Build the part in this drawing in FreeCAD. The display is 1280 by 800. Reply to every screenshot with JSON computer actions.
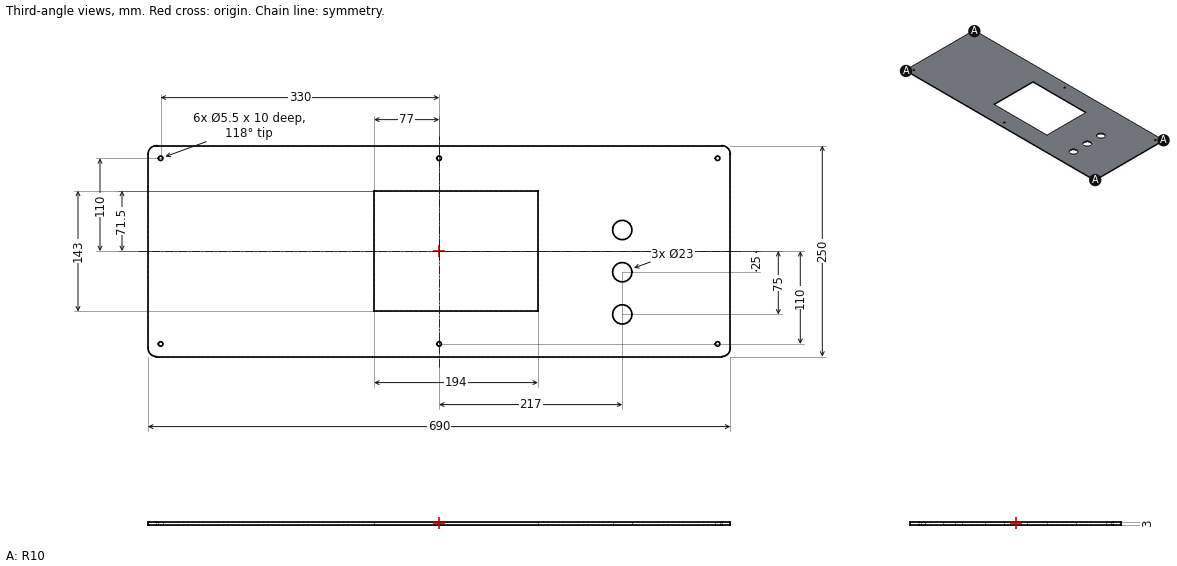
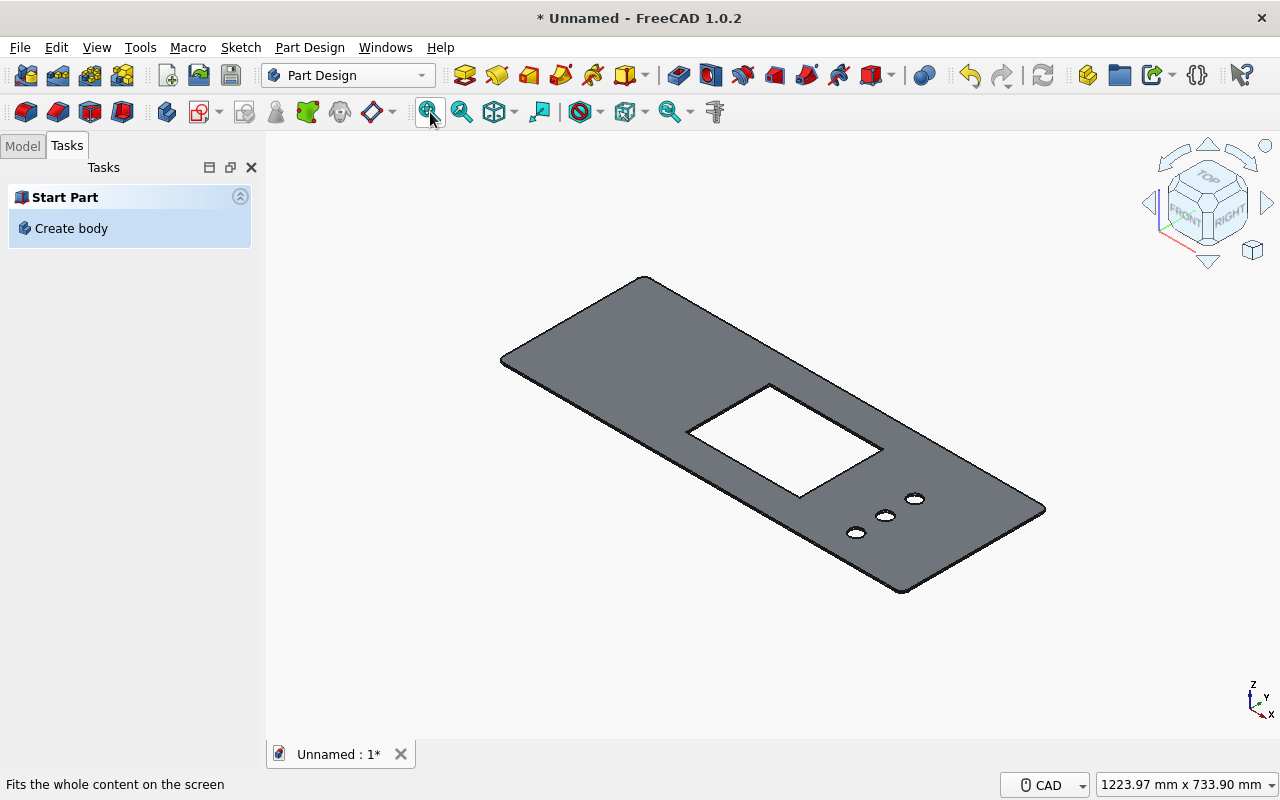
{"action": "left_click", "coordinate": [658, 366]}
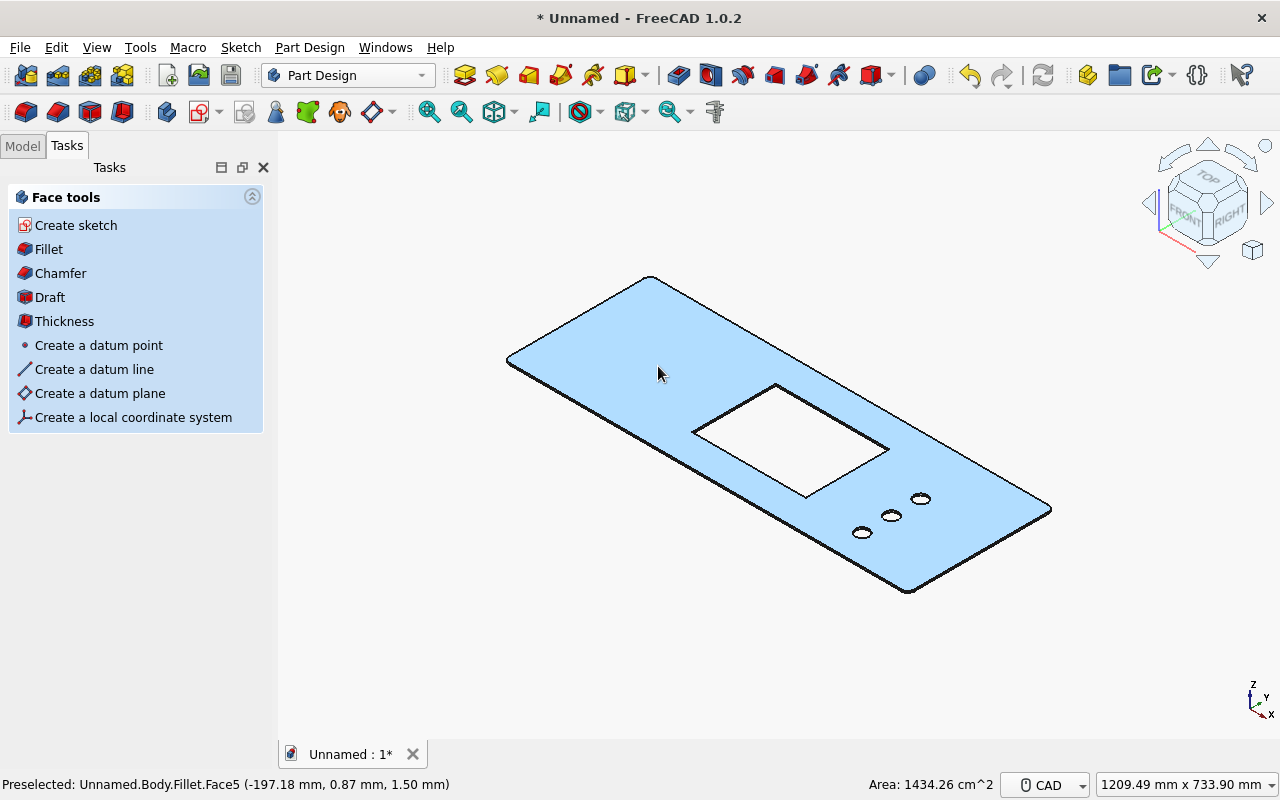
{"action": "left_click", "coordinate": [200, 112]}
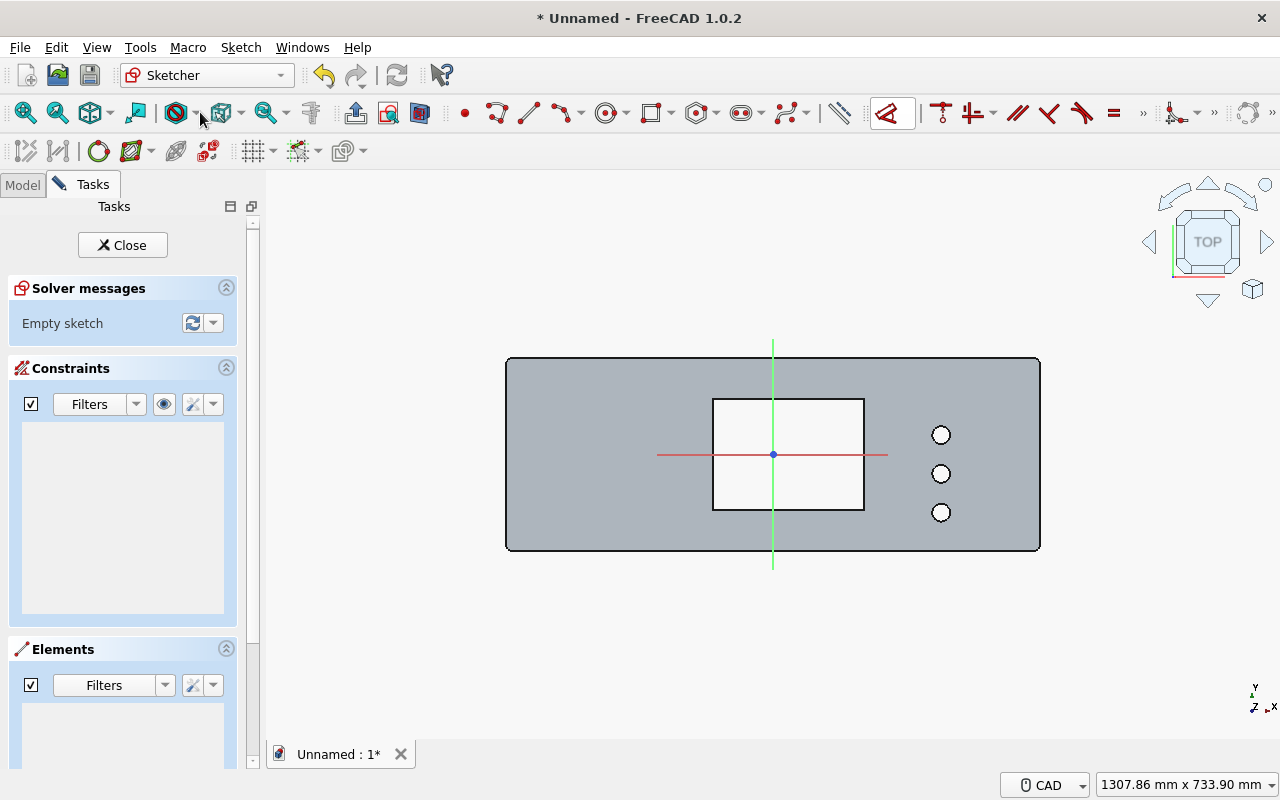
{"action": "left_click", "coordinate": [606, 114]}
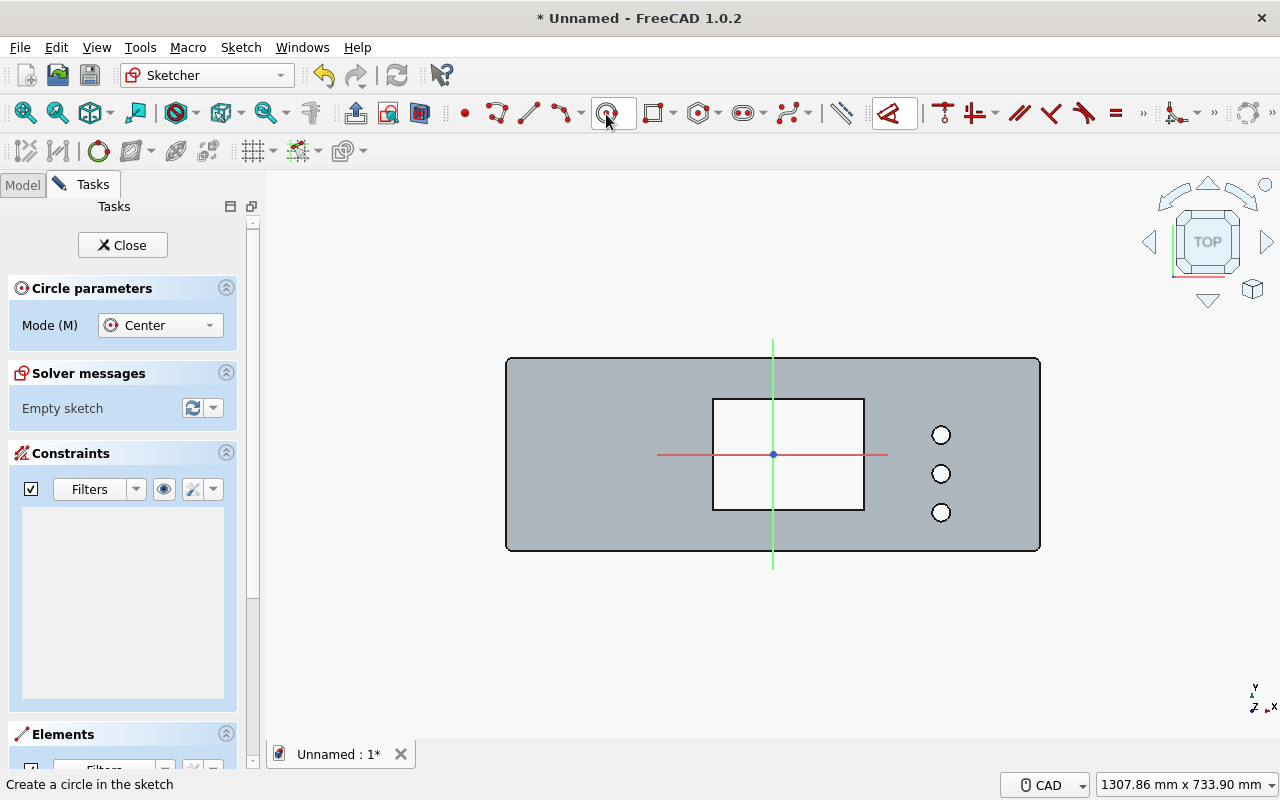
{"action": "scroll", "coordinate": [517, 369], "scroll_direction": "up", "scroll_amount": 12}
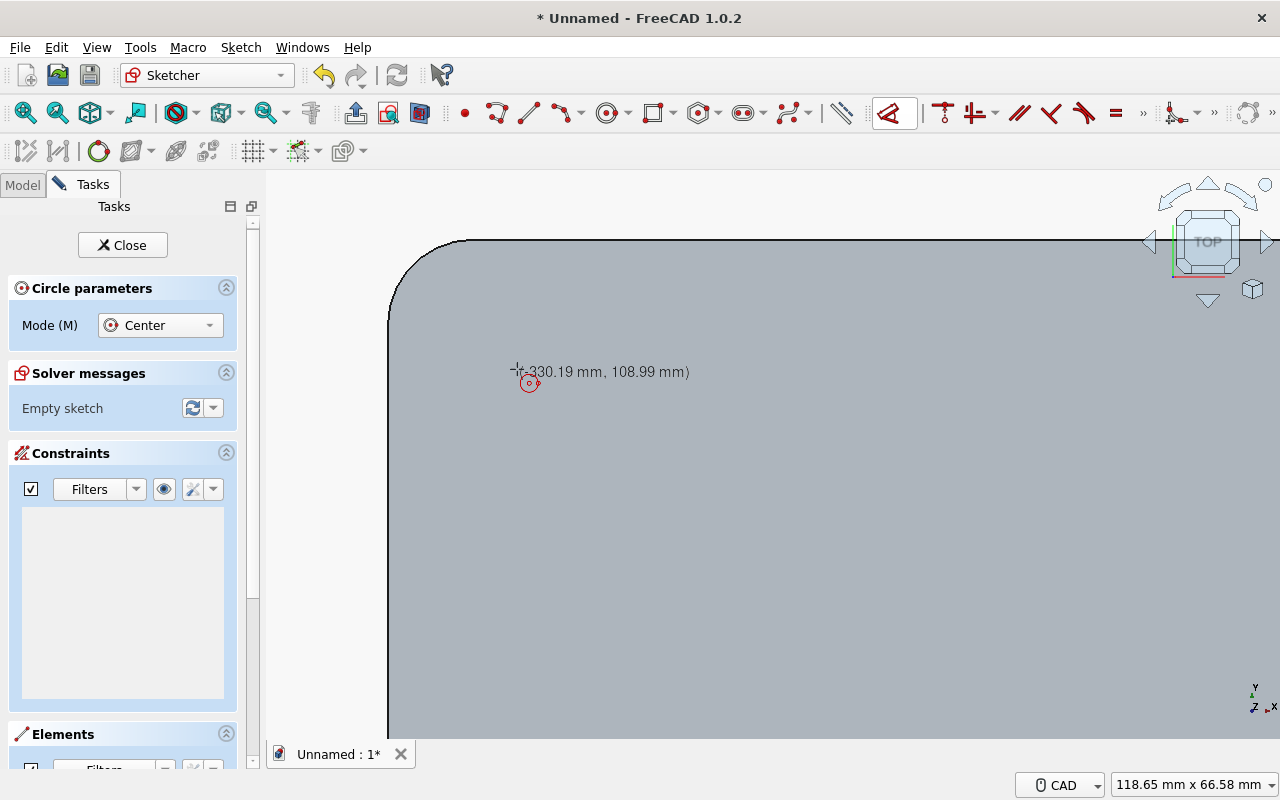
{"action": "scroll", "coordinate": [377, 348], "scroll_direction": "down", "scroll_amount": 11}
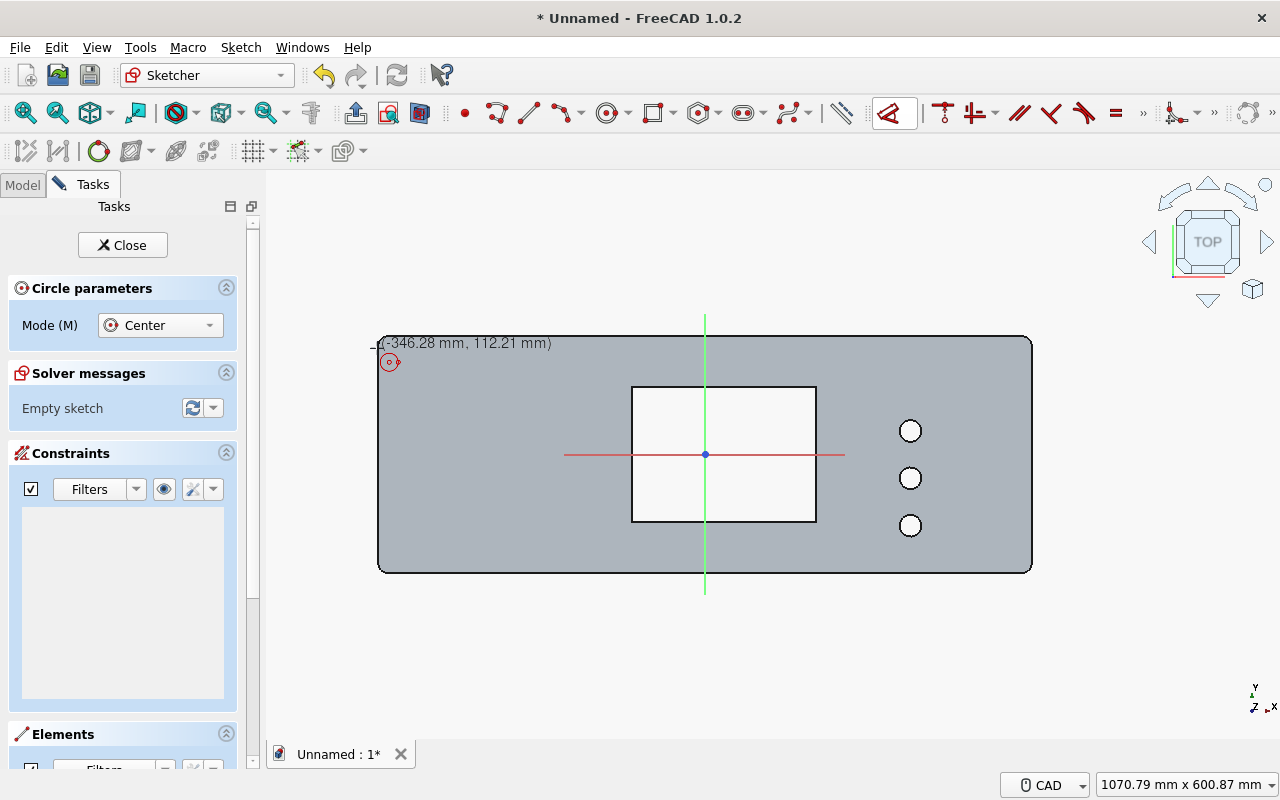
{"action": "left_click", "coordinate": [393, 350]}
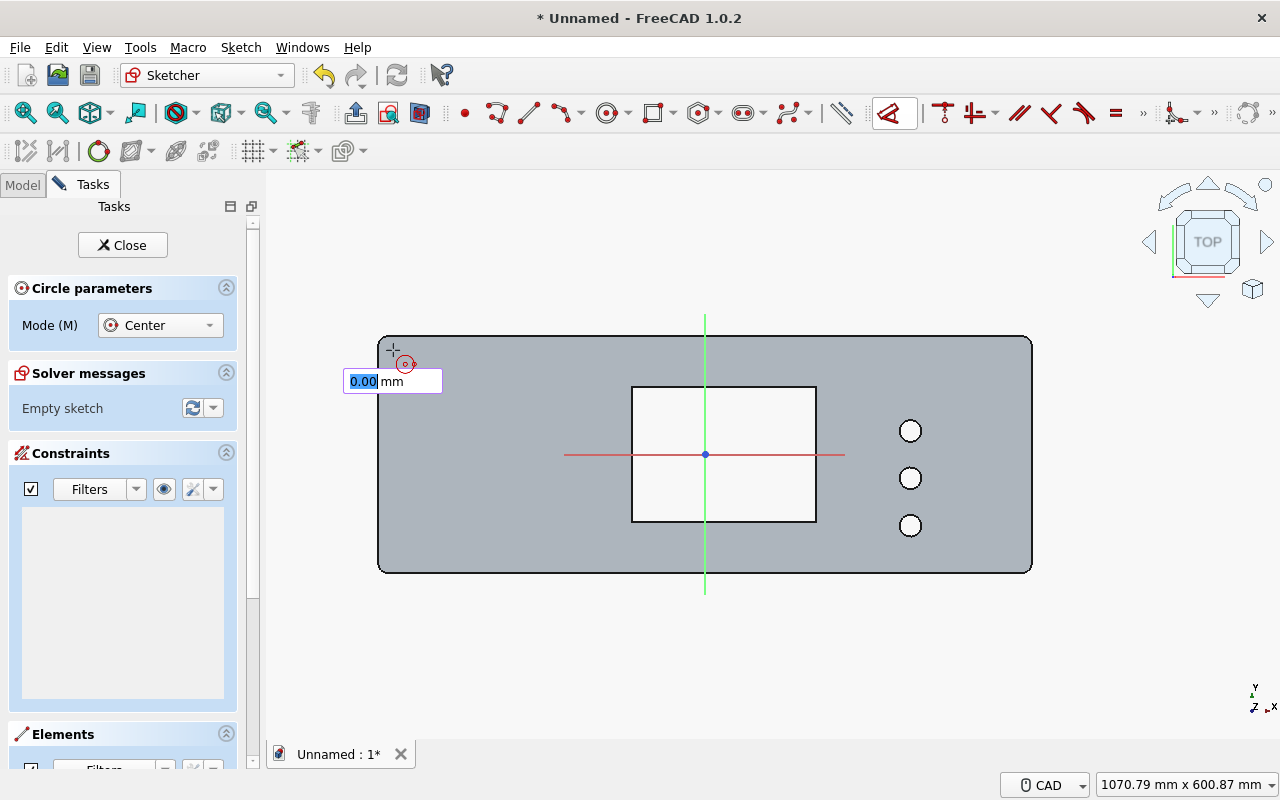
{"action": "scroll", "coordinate": [394, 349], "scroll_direction": "up", "scroll_amount": 10}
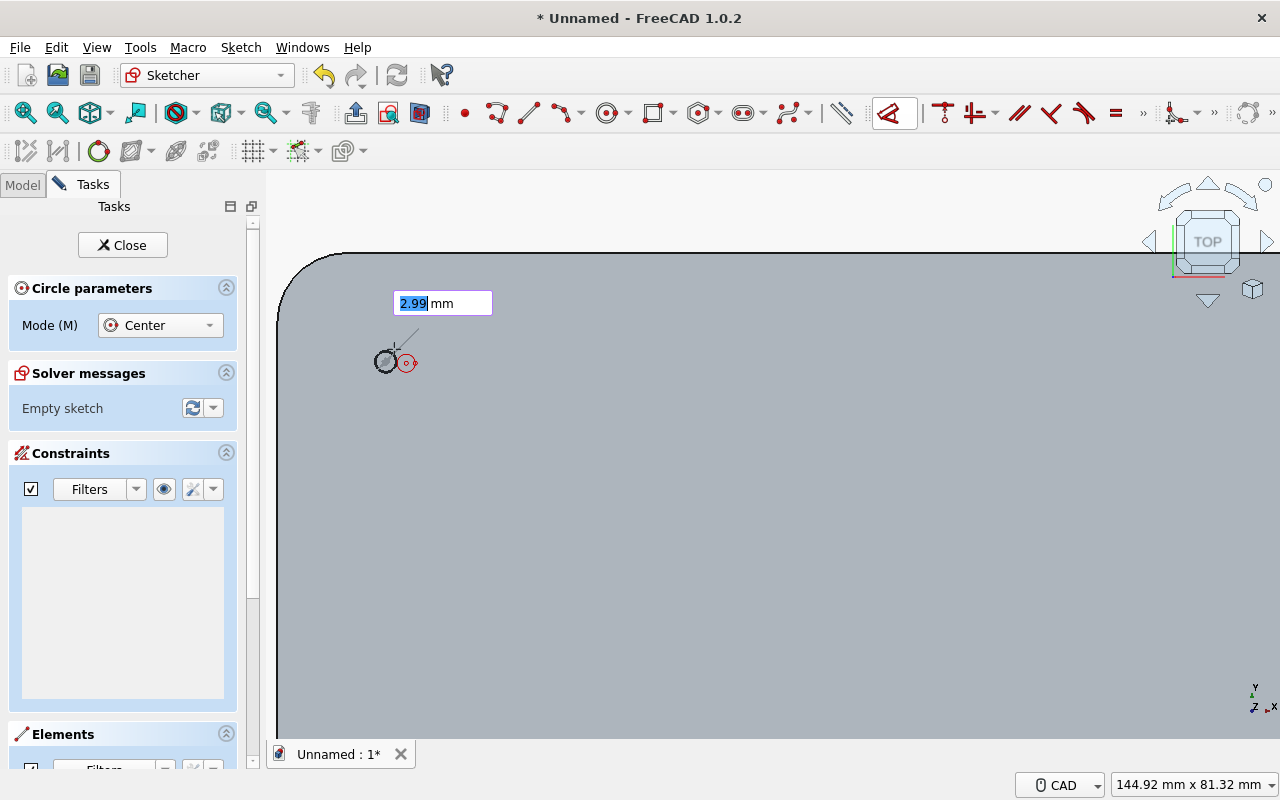
{"action": "left_click", "coordinate": [396, 344]}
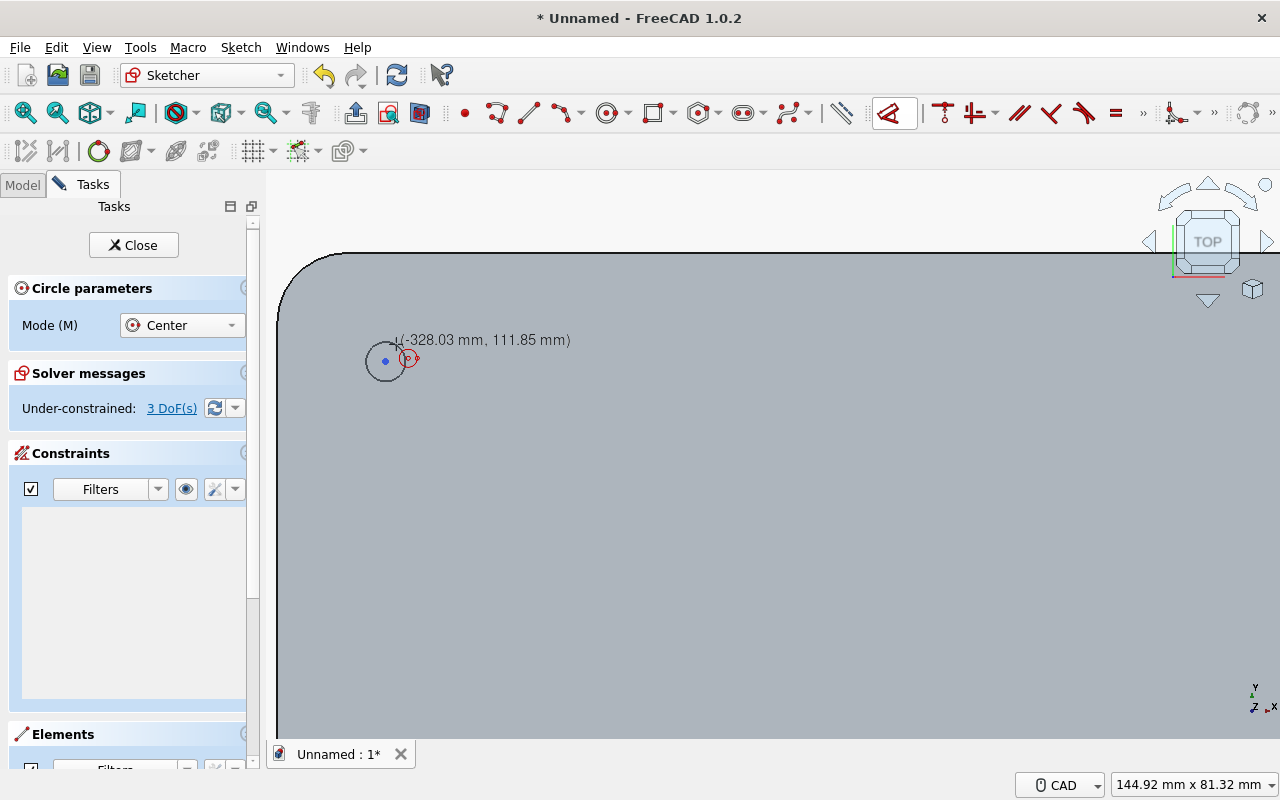
{"action": "scroll", "coordinate": [394, 349], "scroll_direction": "down", "scroll_amount": 10}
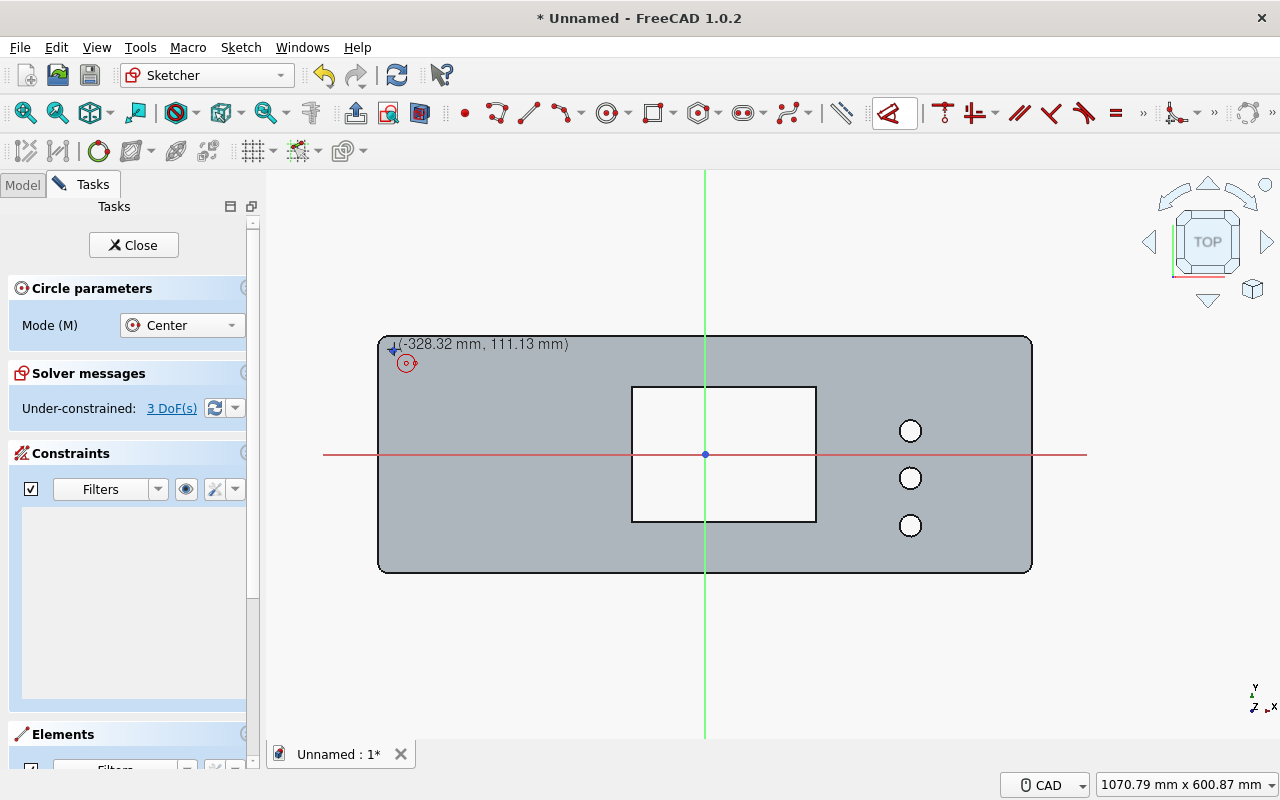
{"action": "scroll", "coordinate": [705, 350], "scroll_direction": "up", "scroll_amount": 11}